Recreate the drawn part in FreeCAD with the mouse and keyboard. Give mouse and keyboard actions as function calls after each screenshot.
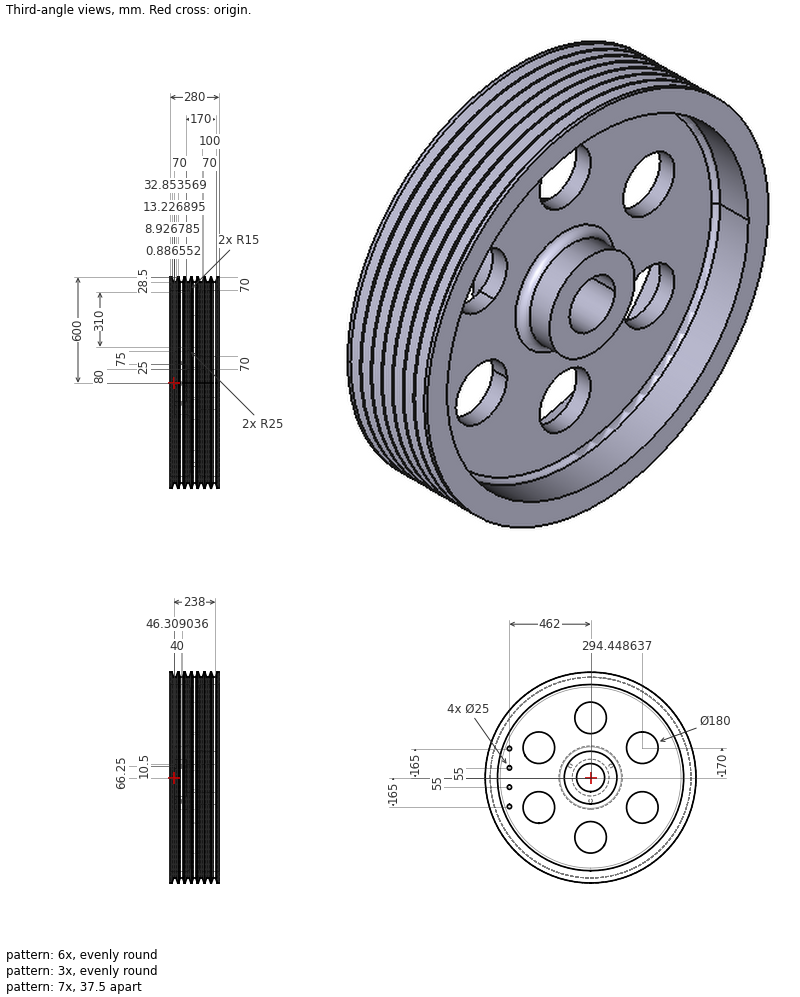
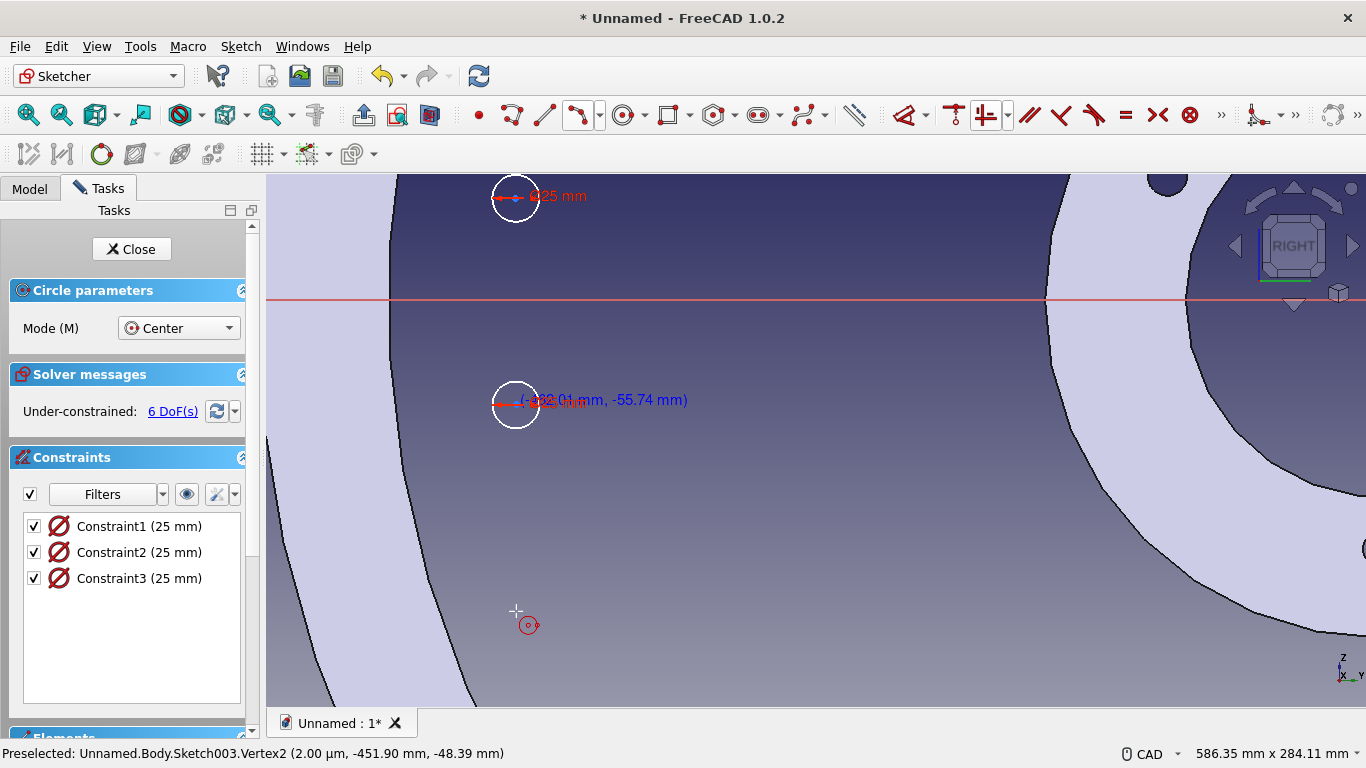
click(516, 610)
move(533, 593)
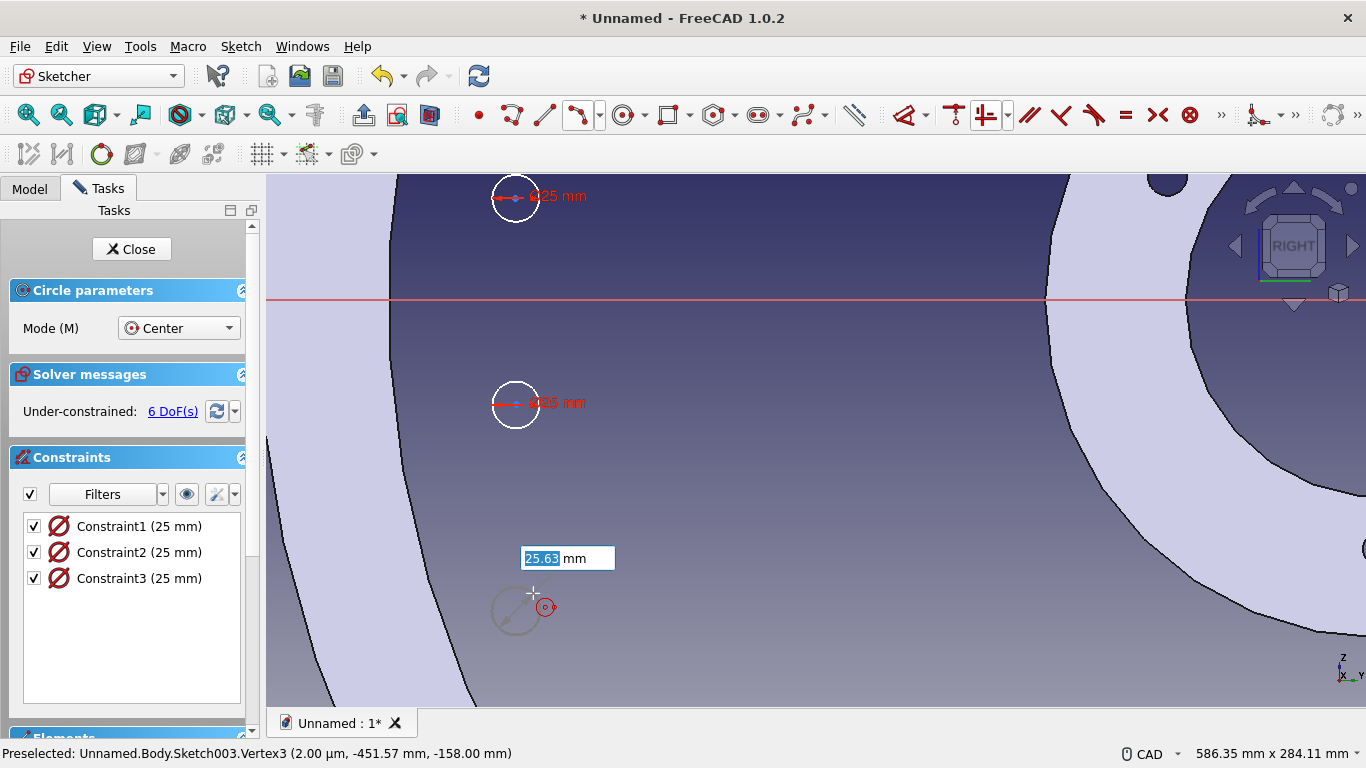
text(25)
key(Return)
key(Escape)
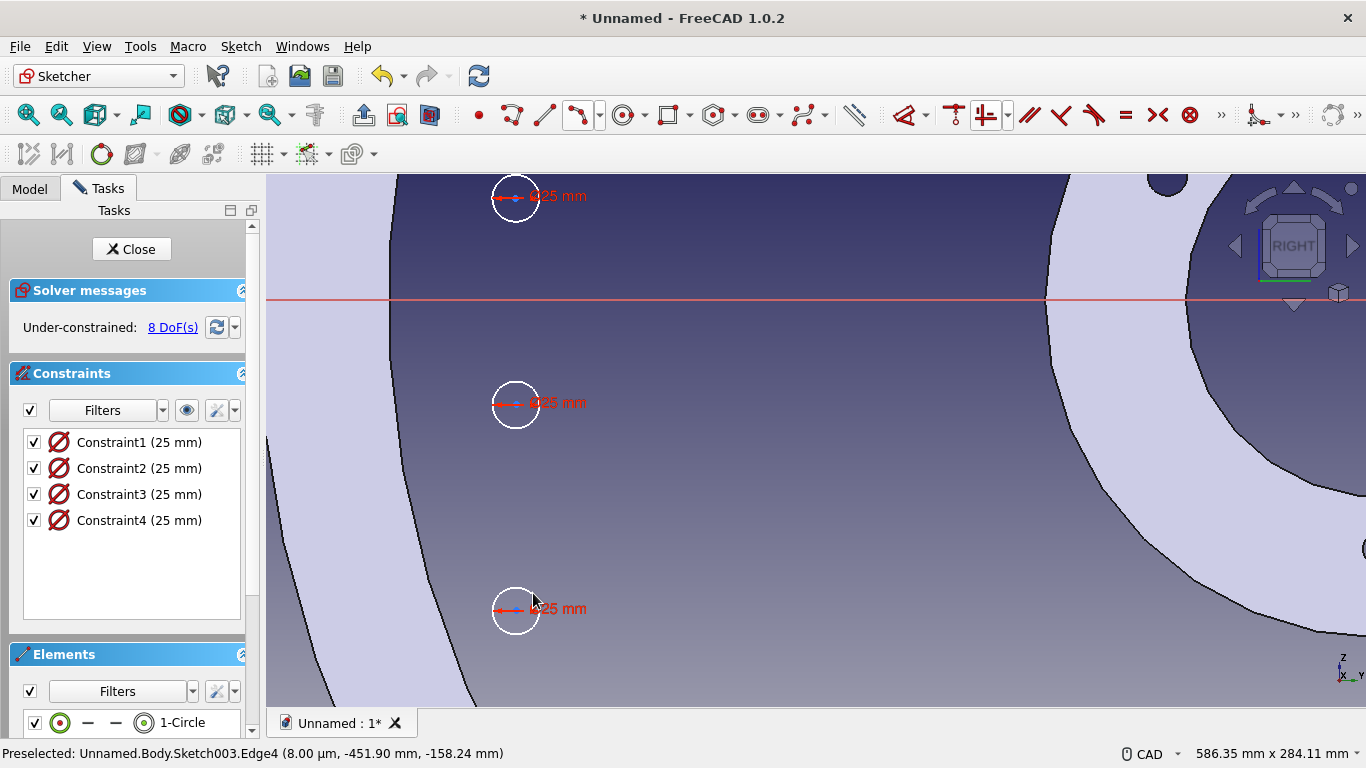
scroll(516, 611, down, 3)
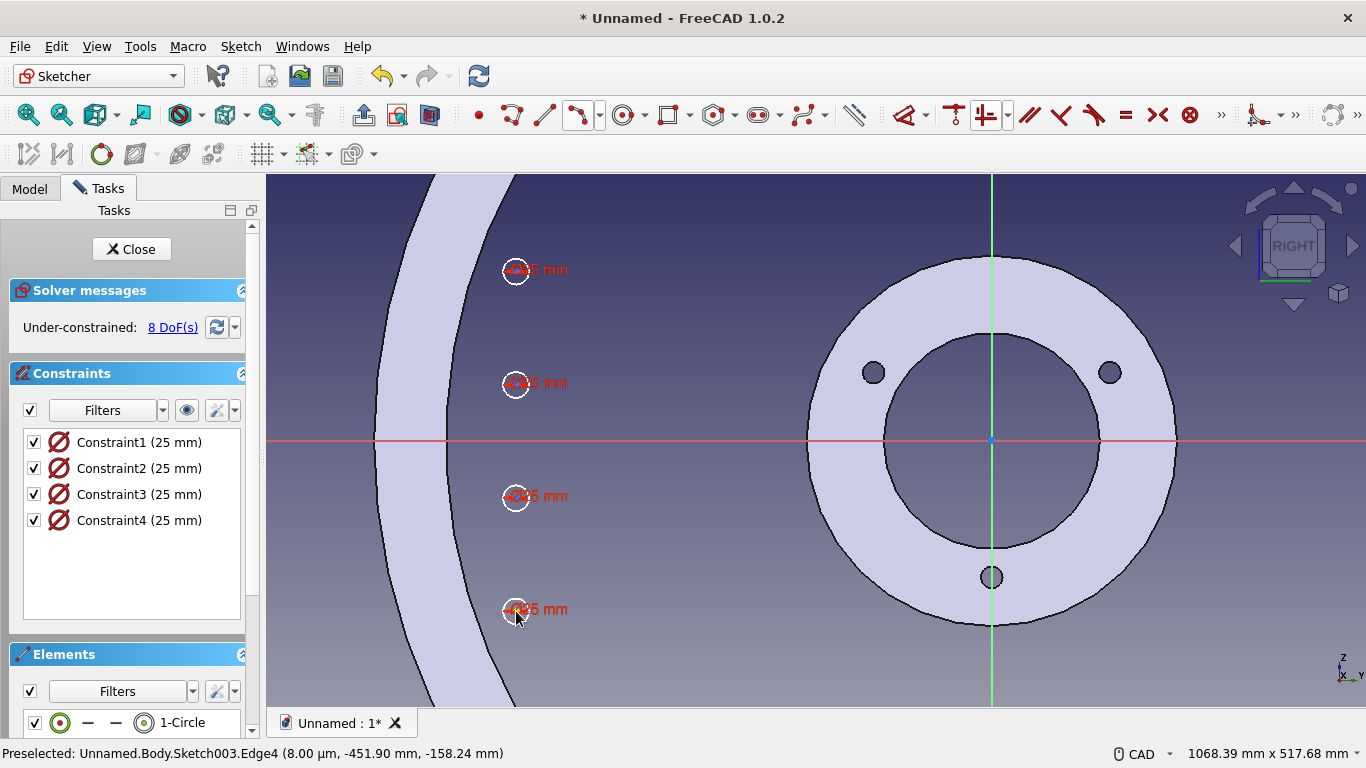
click(516, 385)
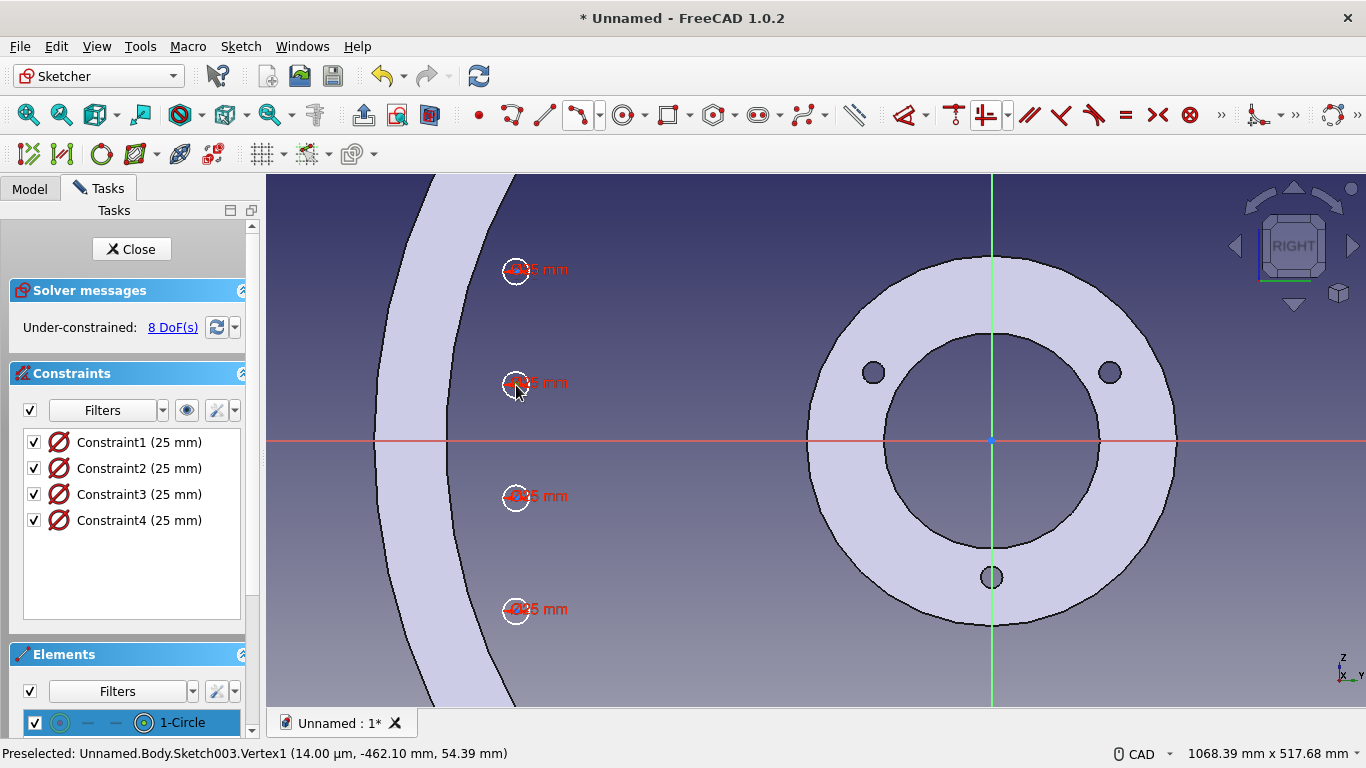
click(516, 272)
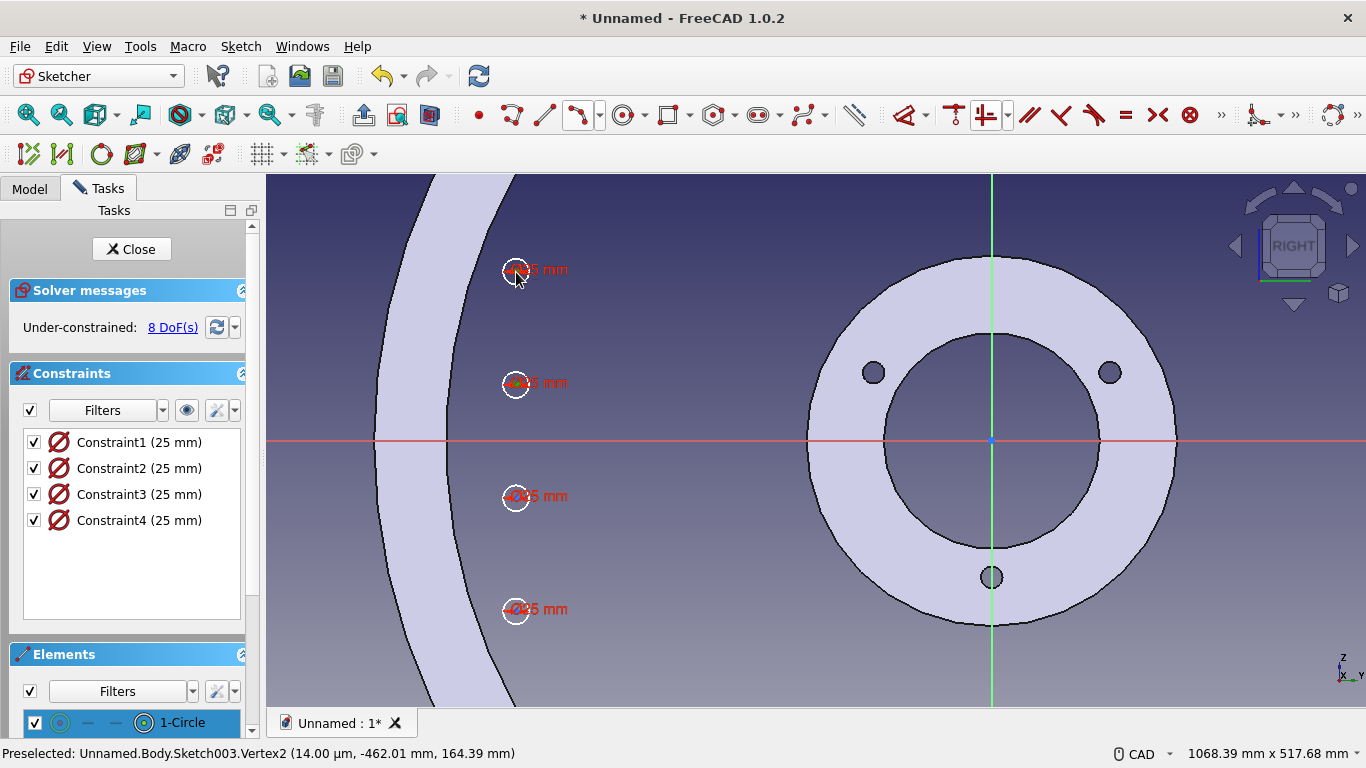
key(v)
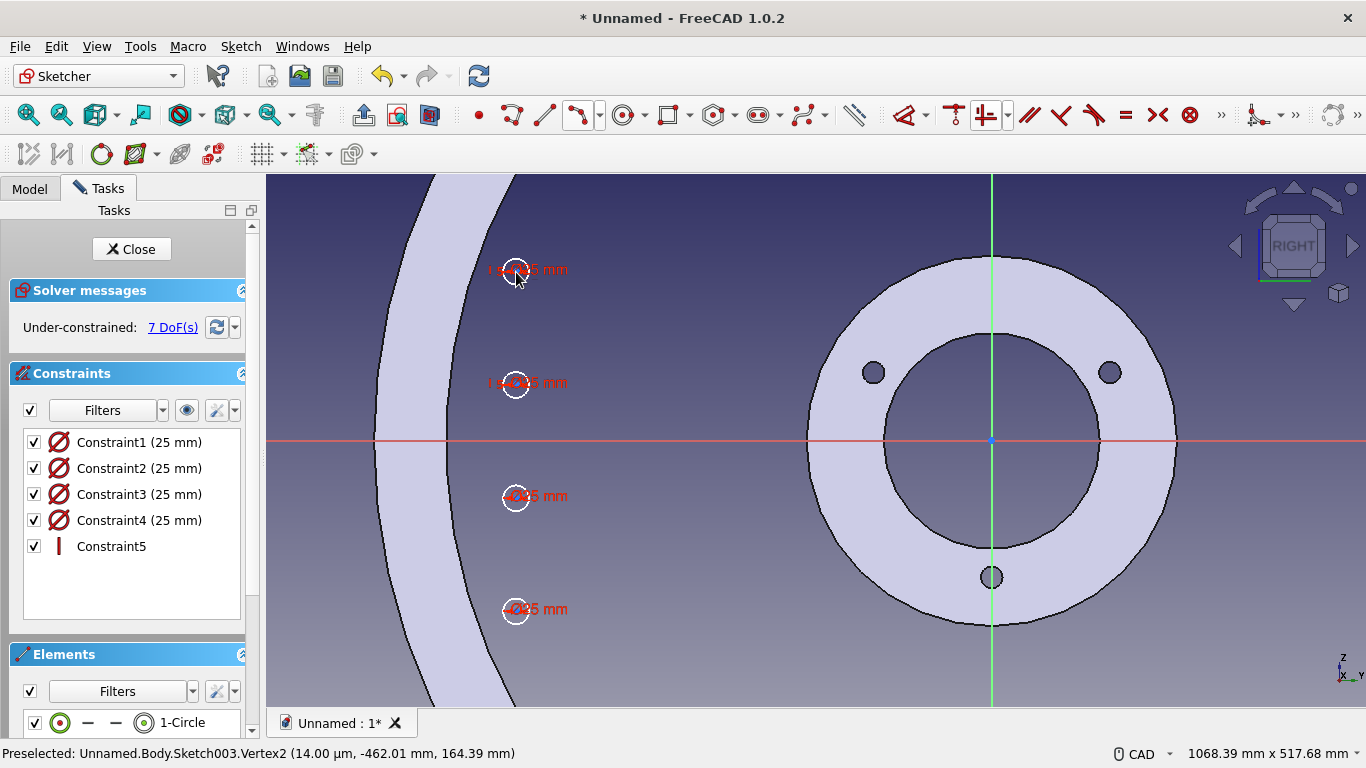
click(516, 385)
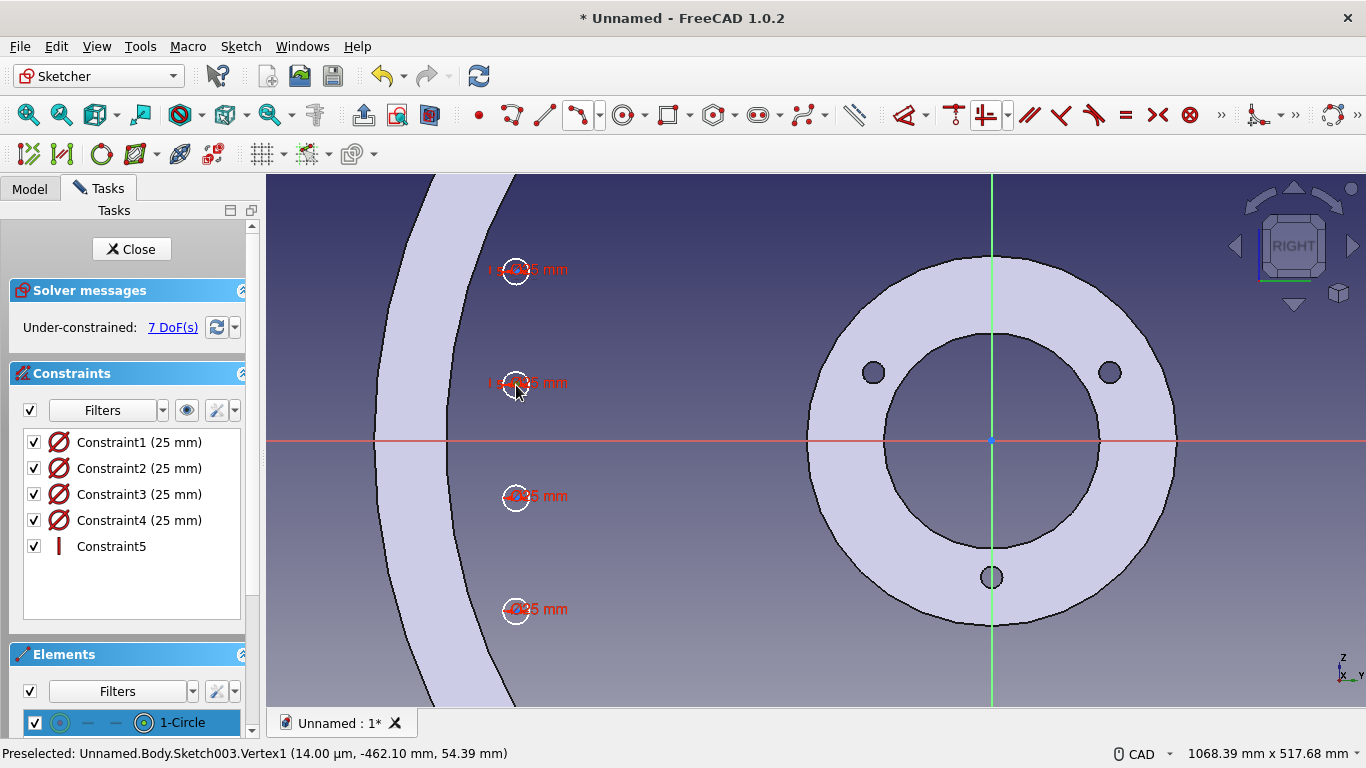
click(516, 498)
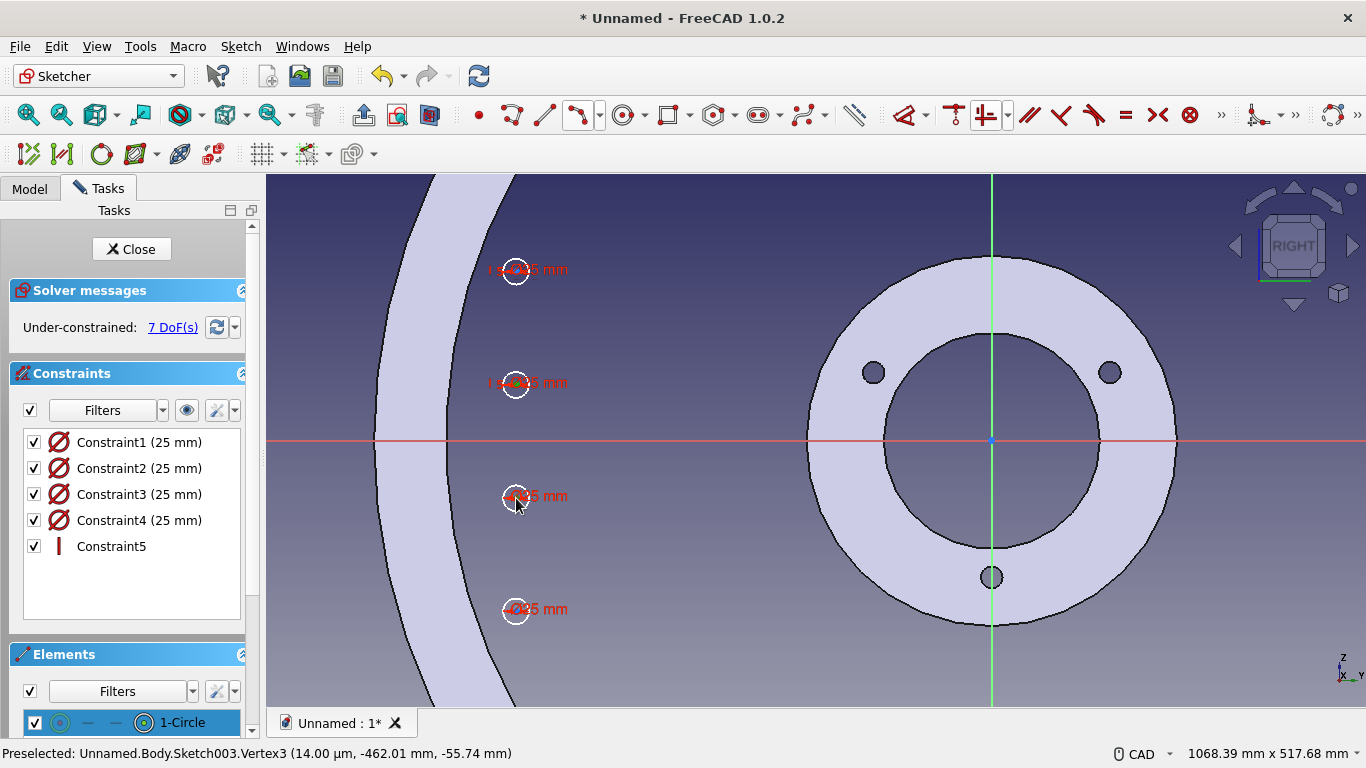
click(1008, 116)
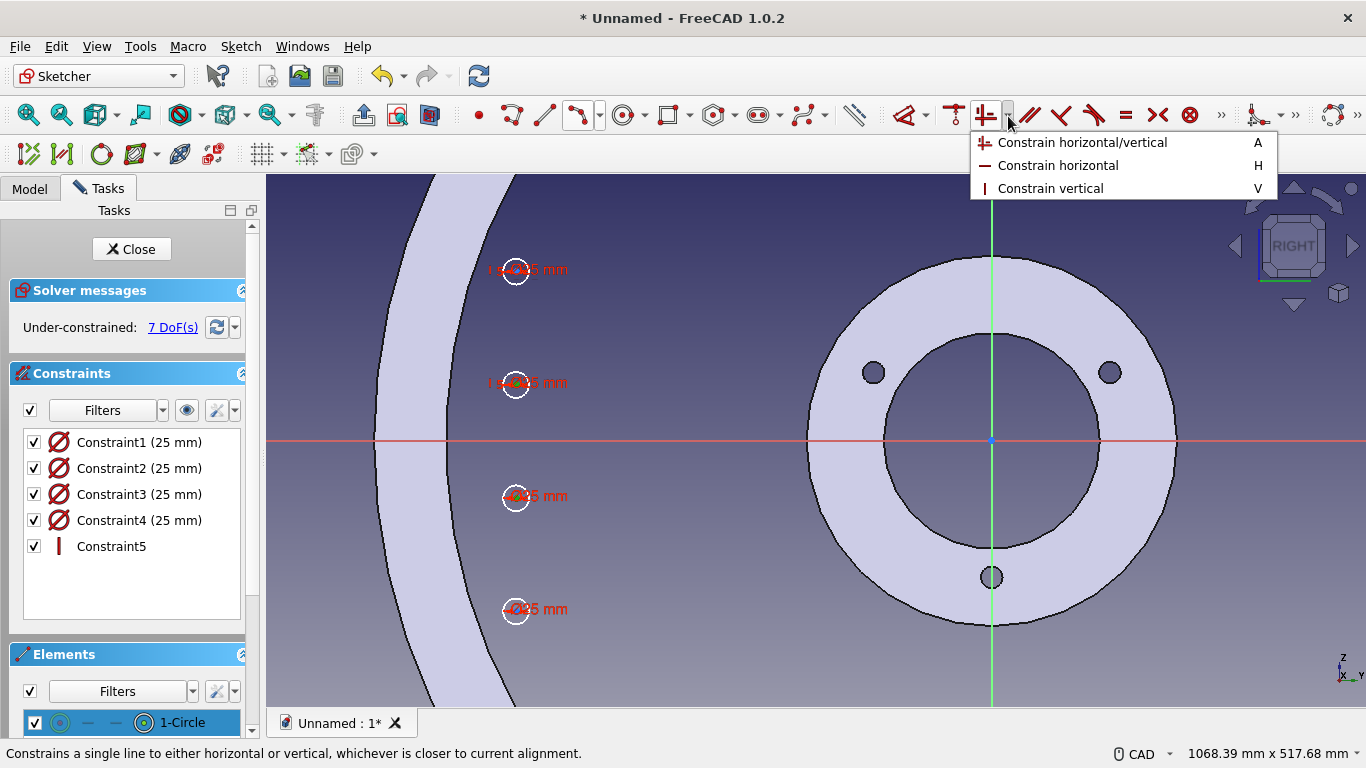
click(1124, 188)